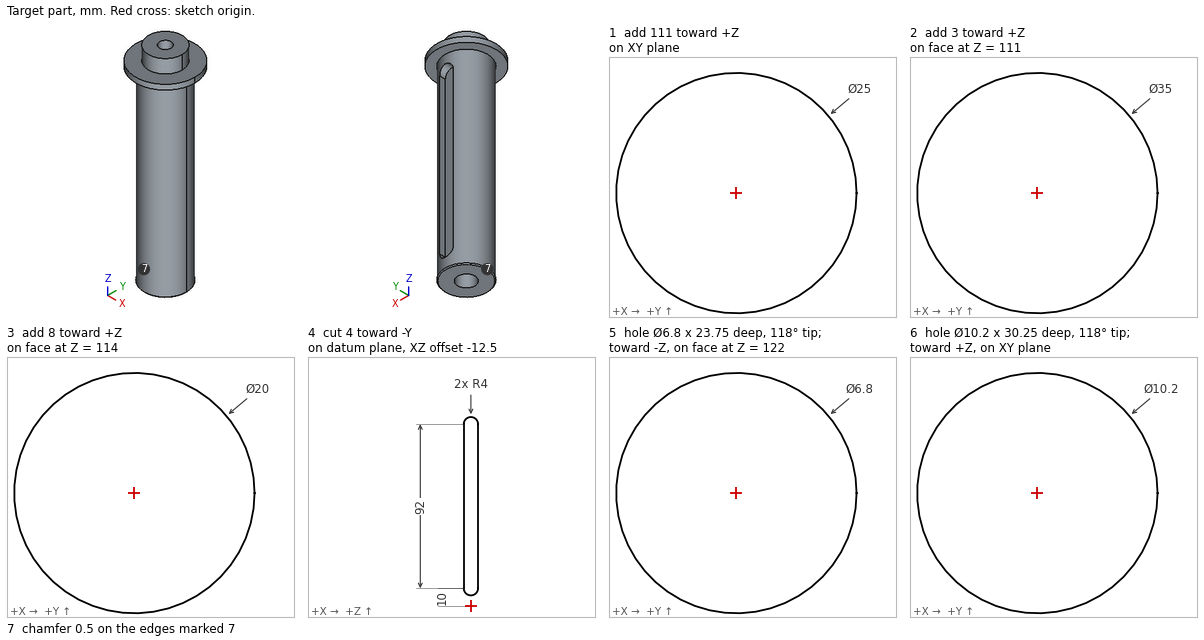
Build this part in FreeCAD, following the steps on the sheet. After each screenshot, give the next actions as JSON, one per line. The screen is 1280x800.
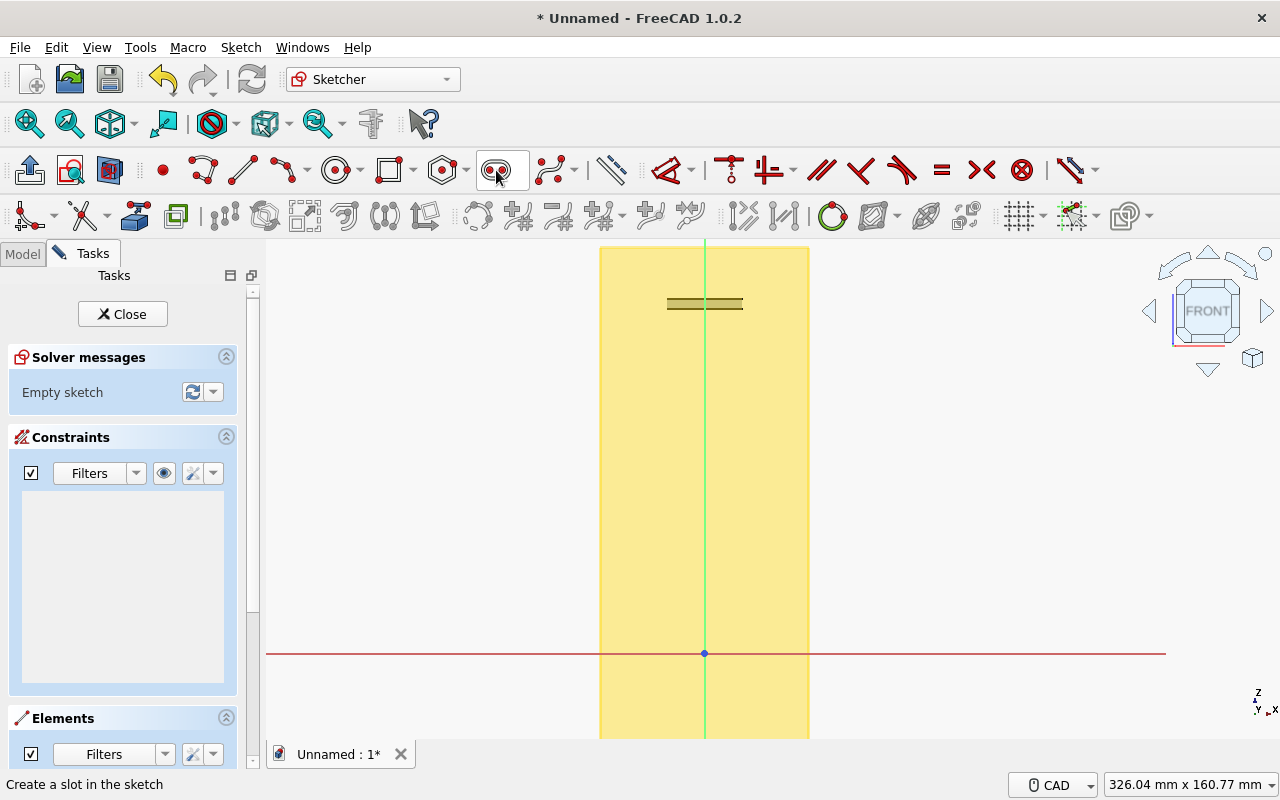
{"action": "scroll", "coordinate": [705, 623], "scroll_direction": "up", "scroll_amount": 4}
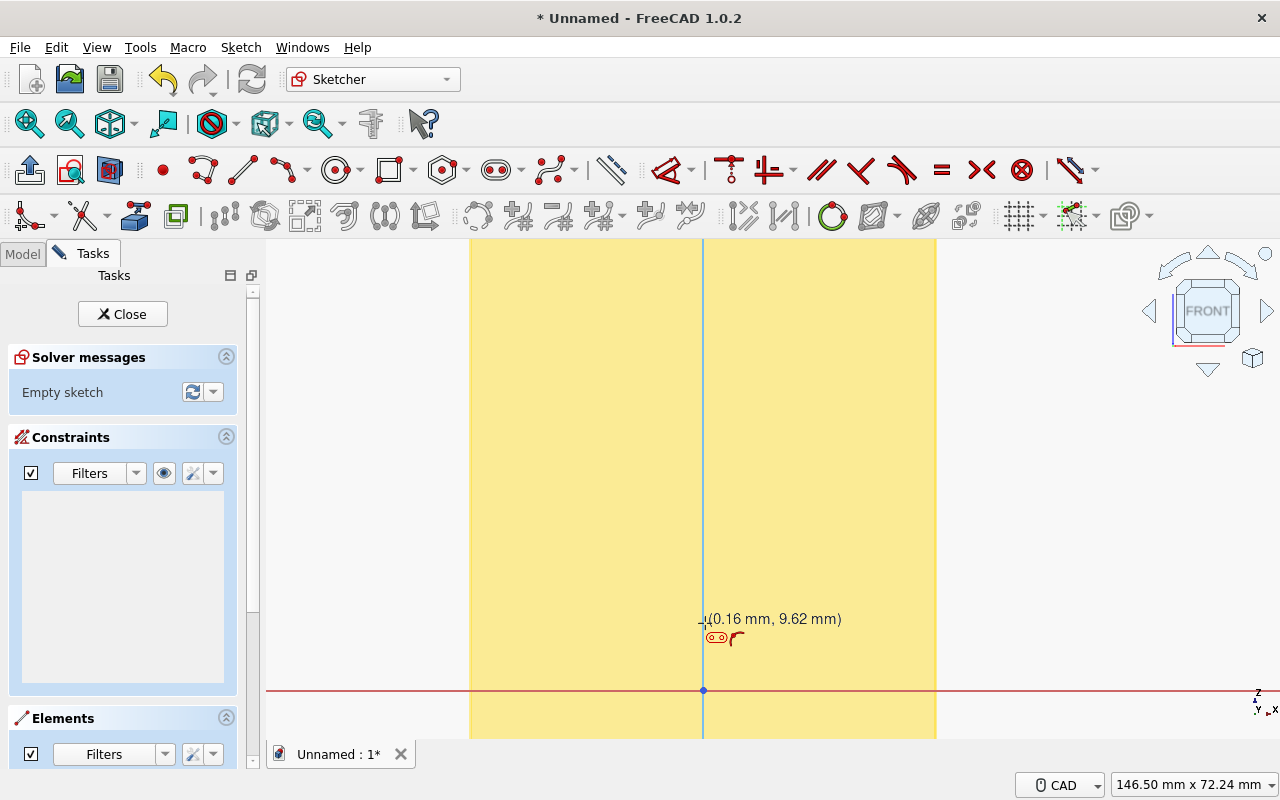
{"action": "left_click", "coordinate": [703, 622]}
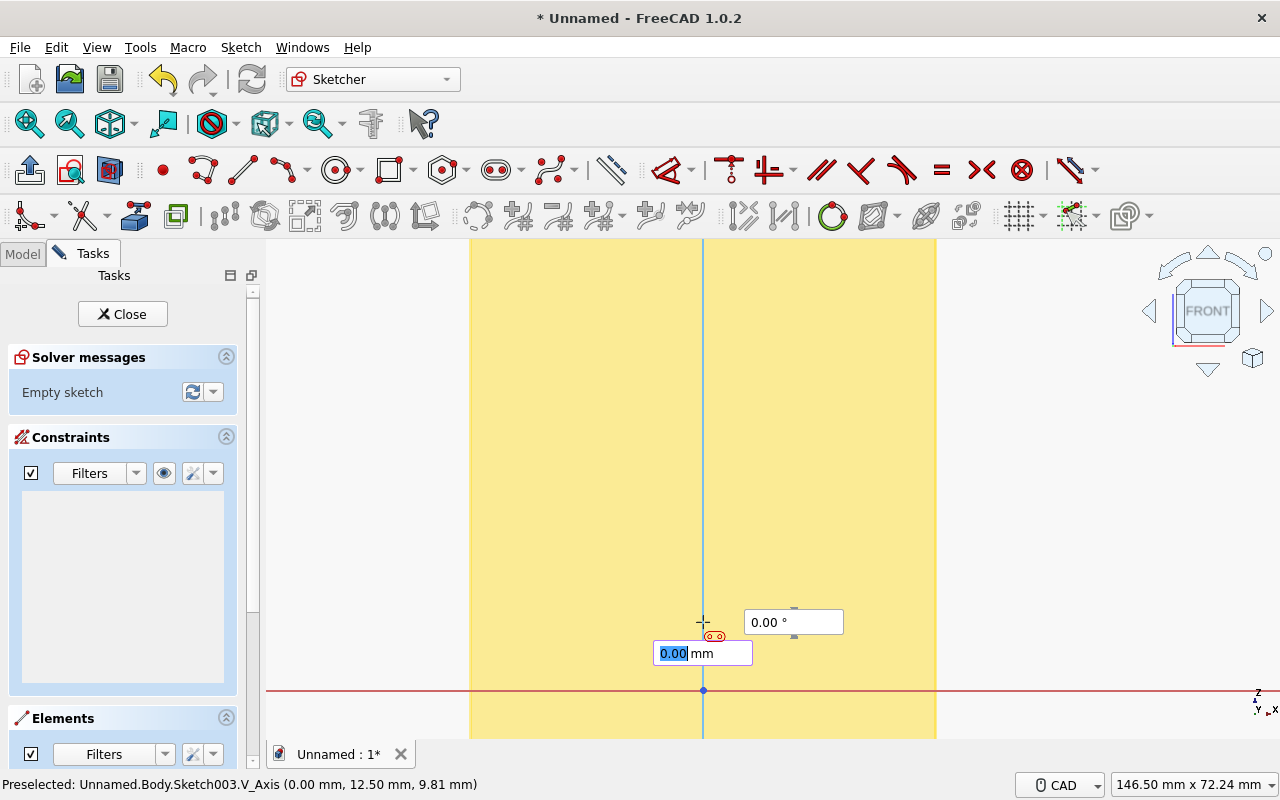
{"action": "scroll", "coordinate": [705, 624], "scroll_direction": "down", "scroll_amount": 4}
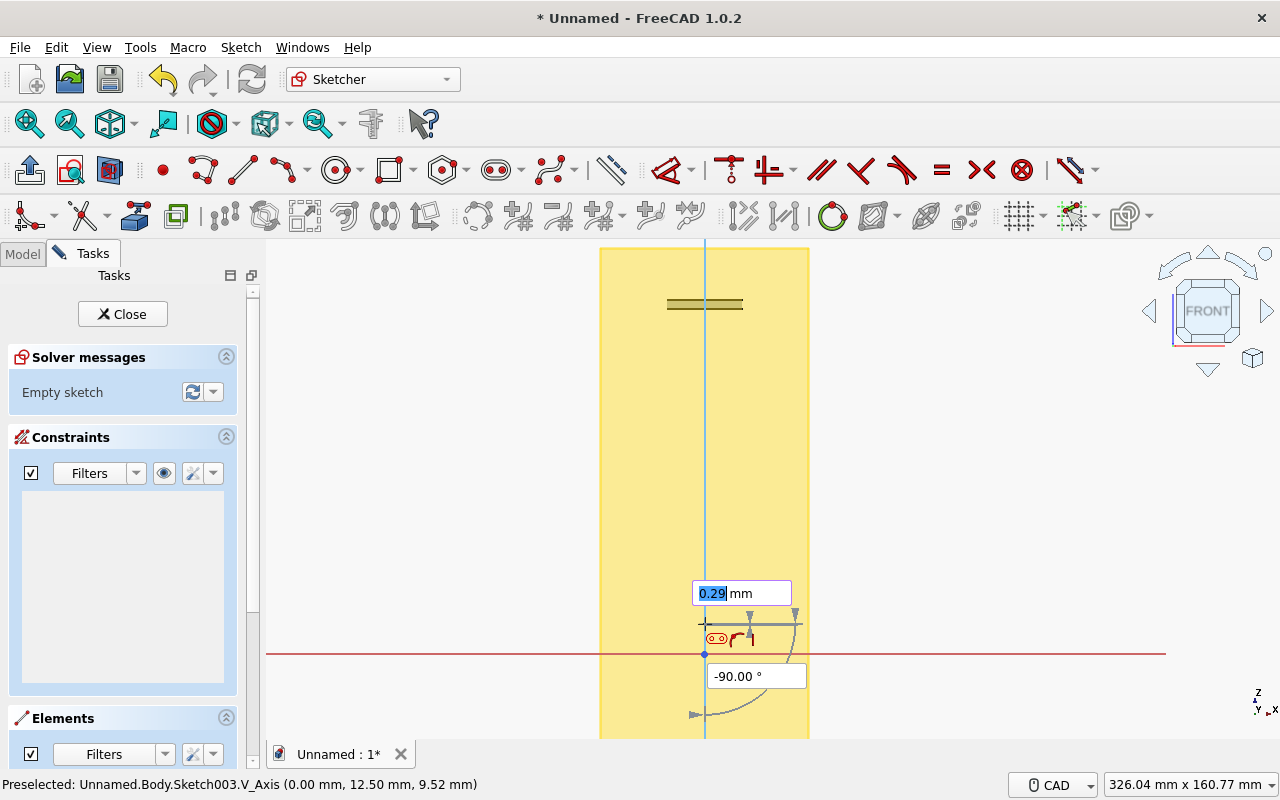
{"action": "left_click", "coordinate": [714, 337]}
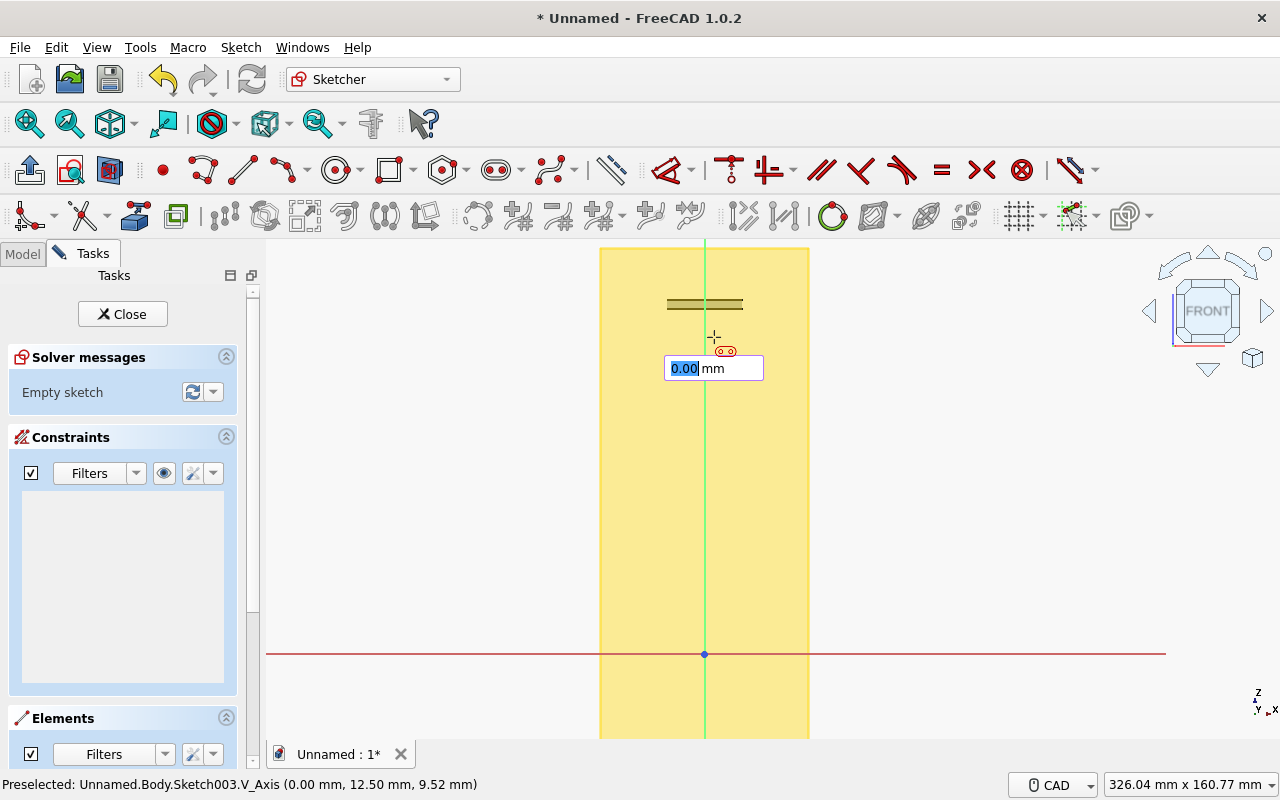
{"action": "scroll", "coordinate": [717, 480], "scroll_direction": "up", "scroll_amount": 2}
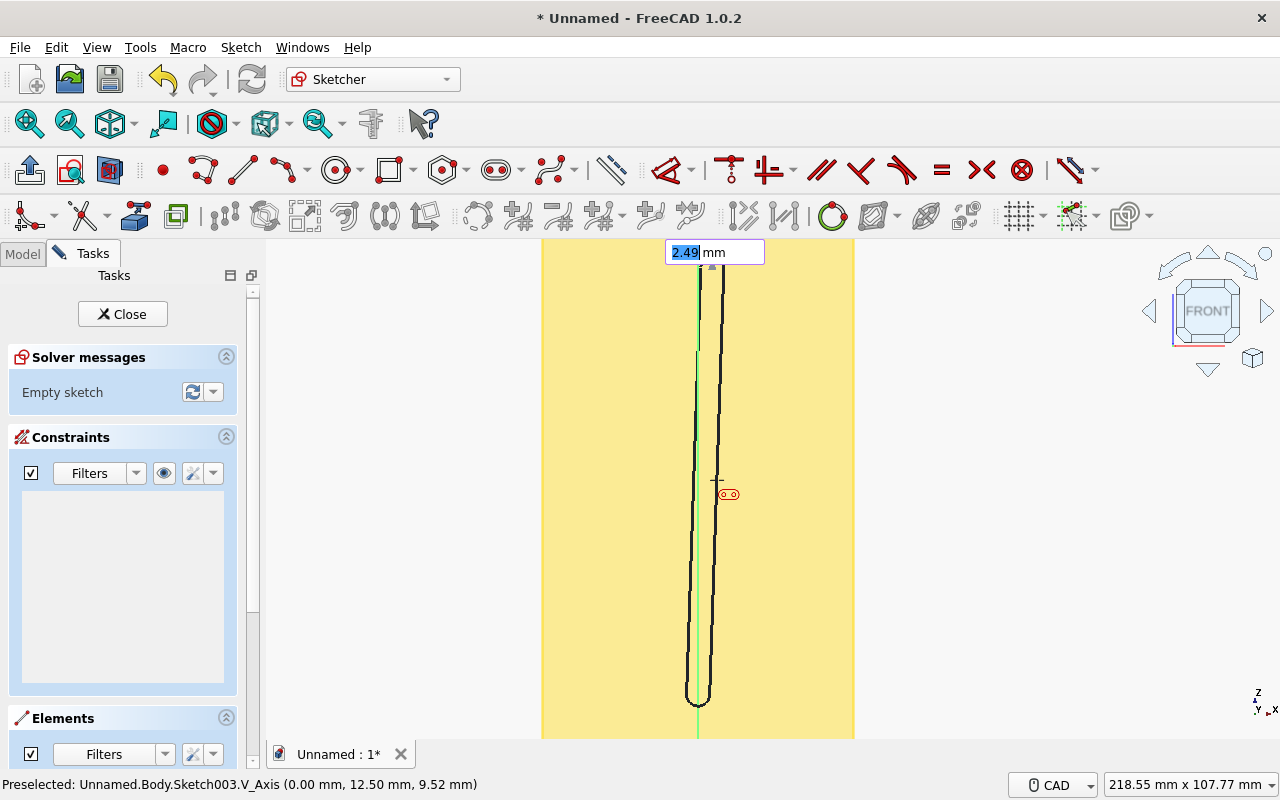
{"action": "left_click", "coordinate": [717, 480]}
{"action": "key", "text": "Escape"}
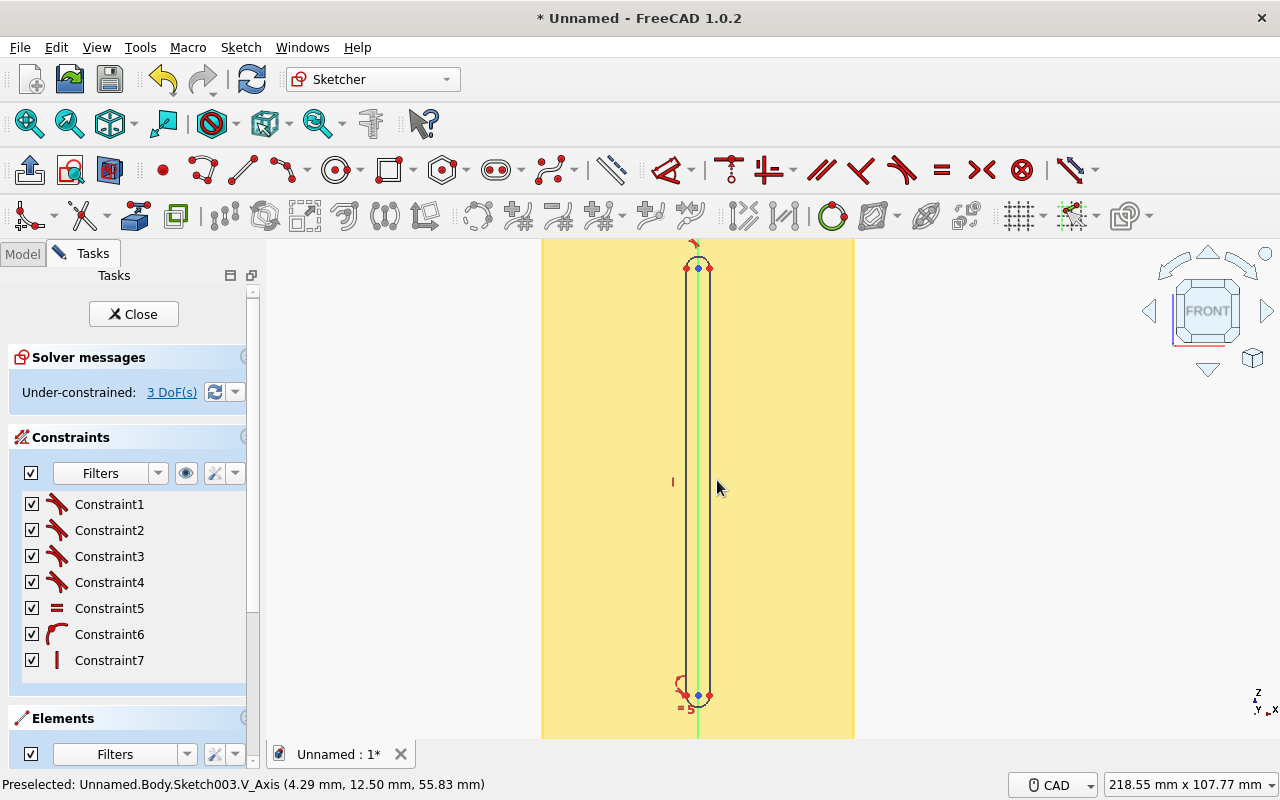
{"action": "left_click", "coordinate": [666, 170]}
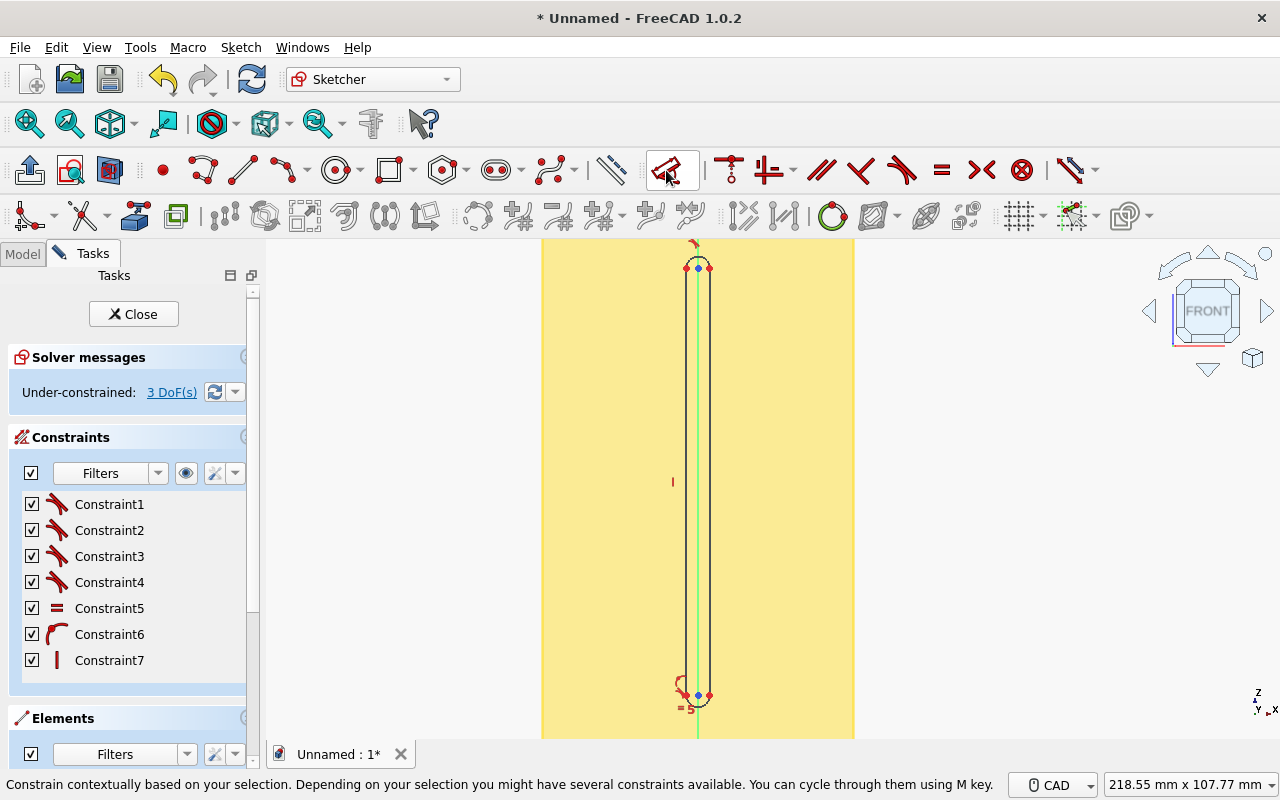
{"action": "scroll", "coordinate": [698, 707], "scroll_direction": "up", "scroll_amount": 4}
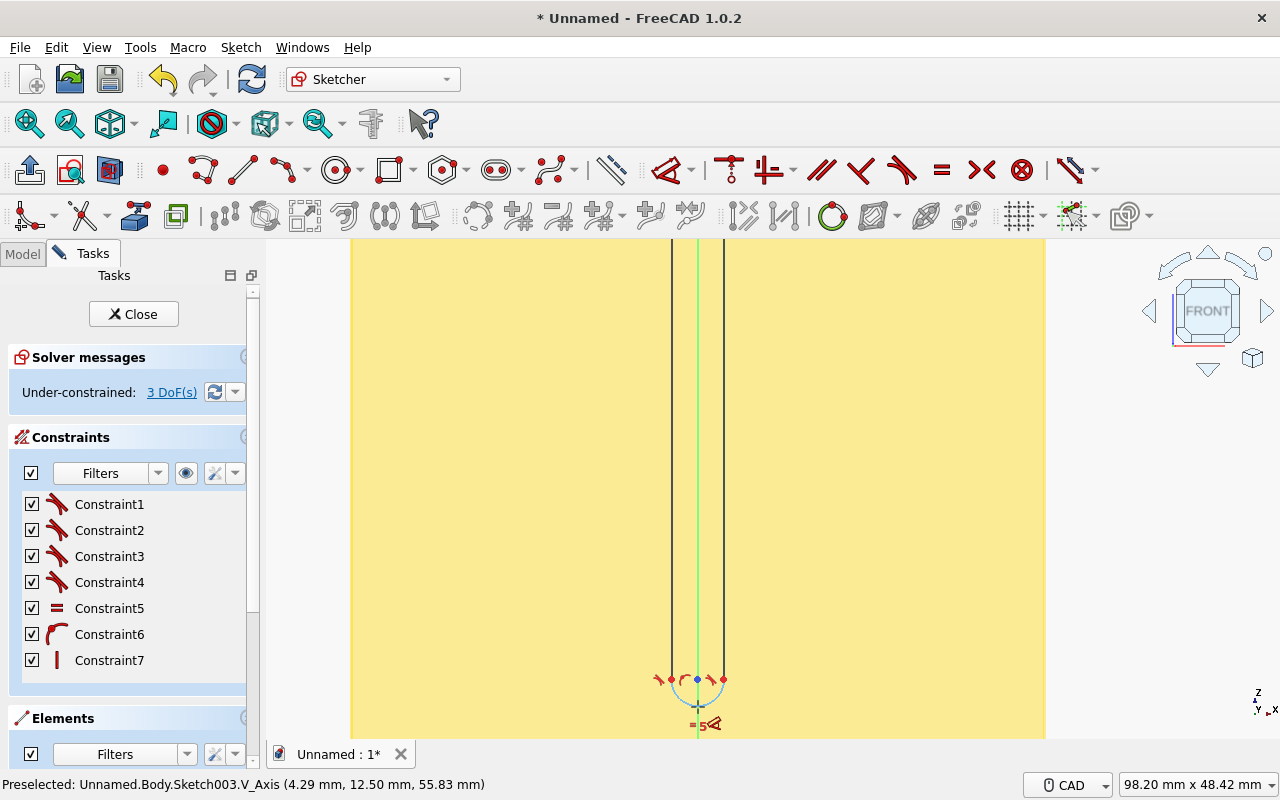
{"action": "left_click", "coordinate": [698, 706]}
{"action": "left_click", "coordinate": [747, 711]}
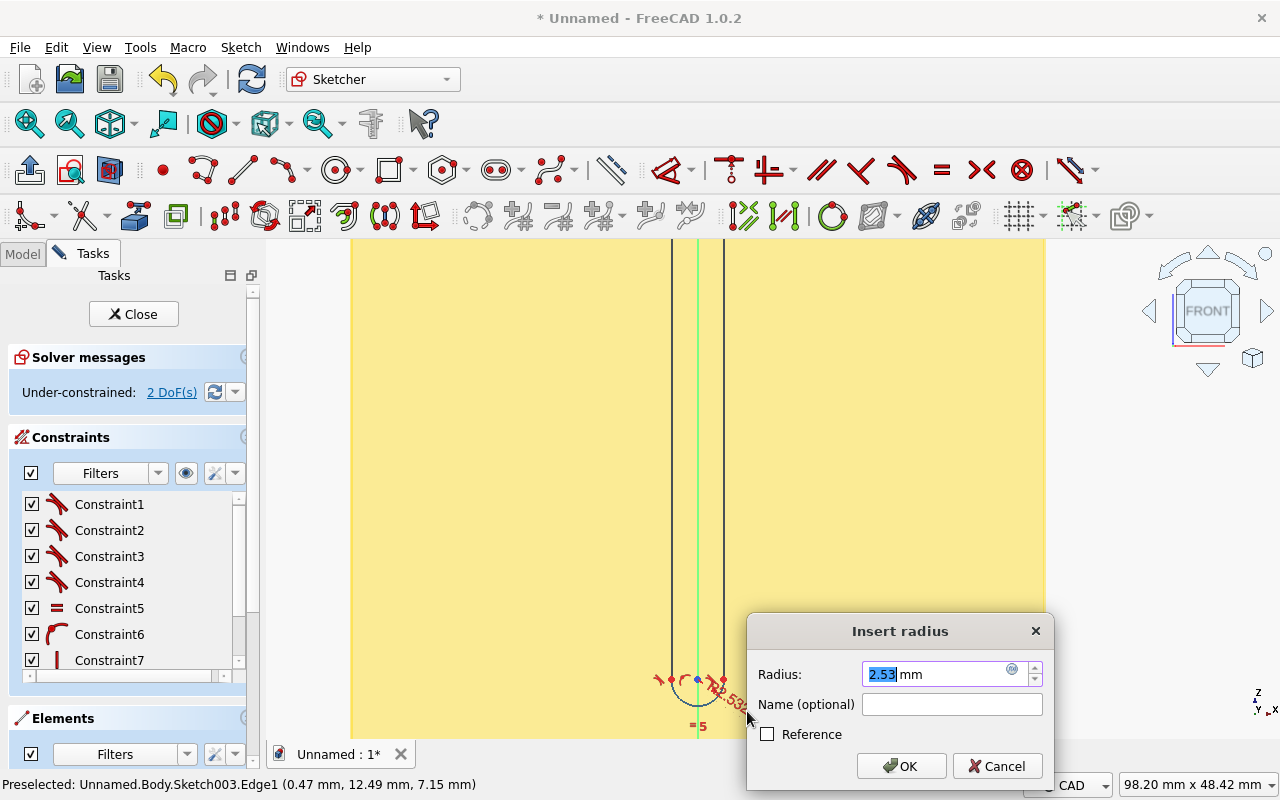
{"action": "type", "text": "4"}
{"action": "key", "text": "Return"}